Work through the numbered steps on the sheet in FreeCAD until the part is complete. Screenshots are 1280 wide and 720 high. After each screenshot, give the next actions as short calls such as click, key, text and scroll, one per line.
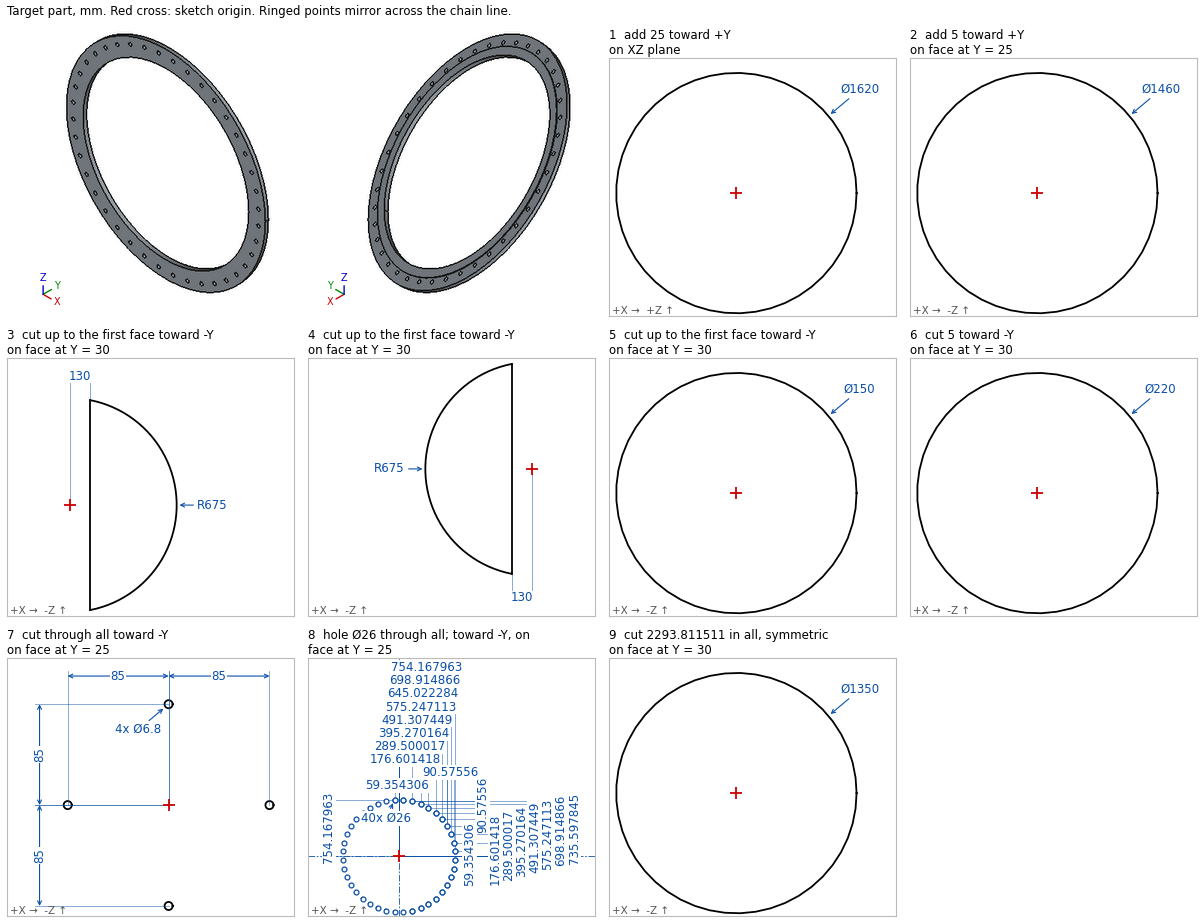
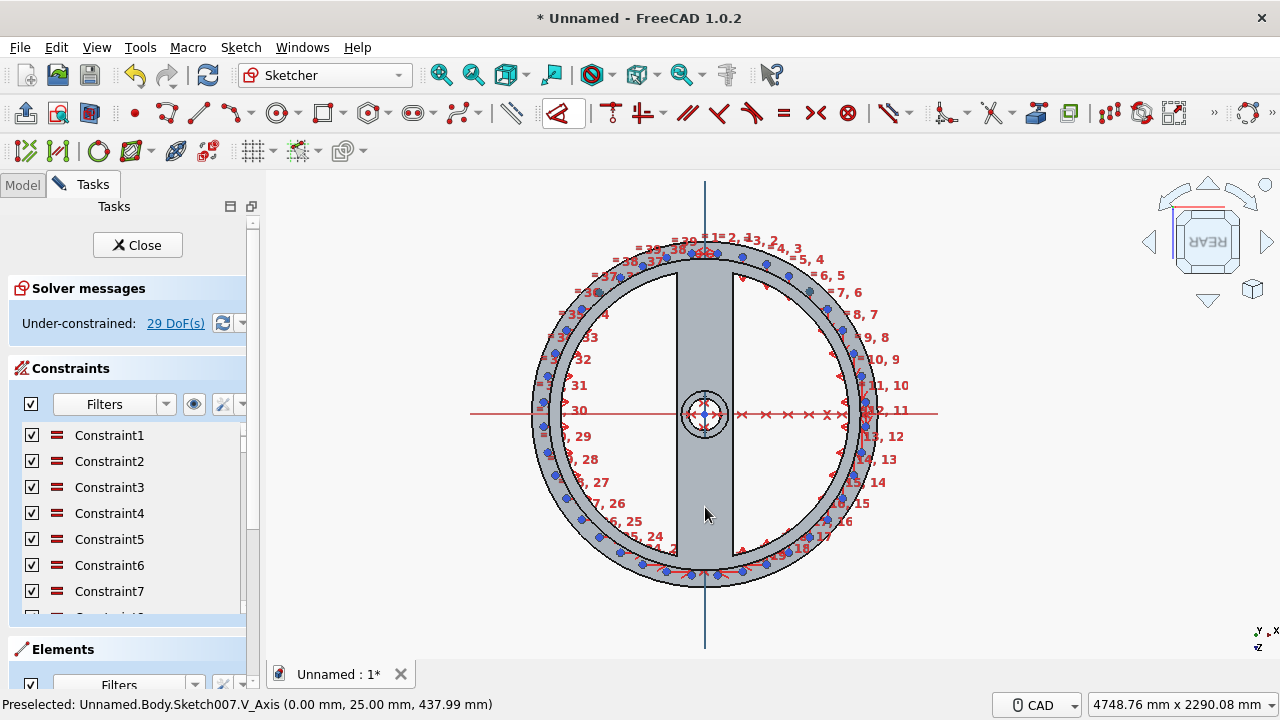
click(816, 114)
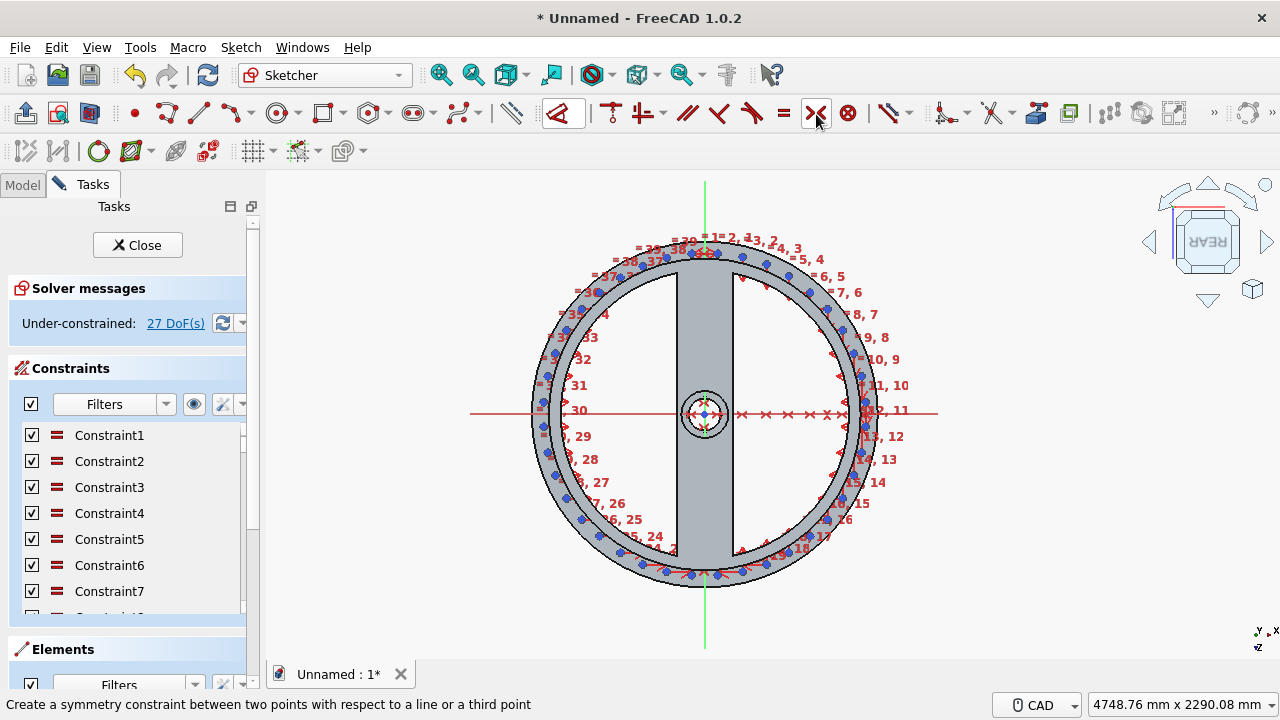
click(789, 276)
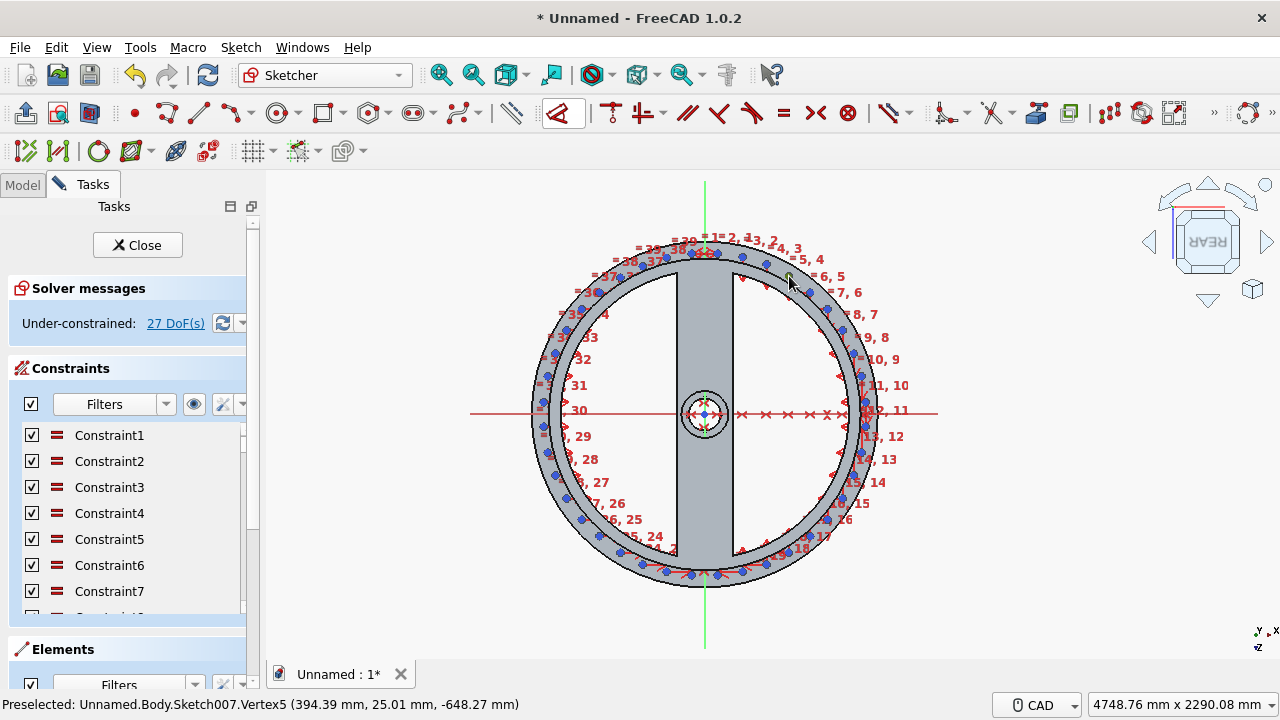
click(620, 278)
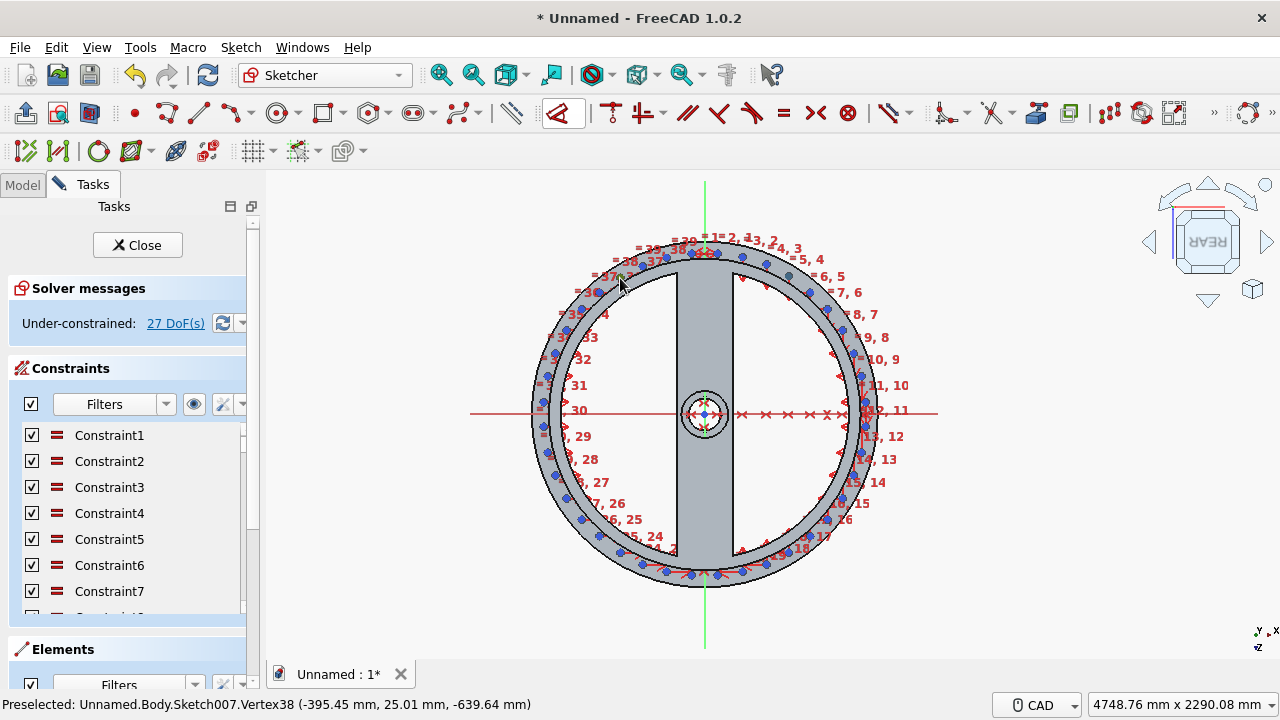
click(705, 507)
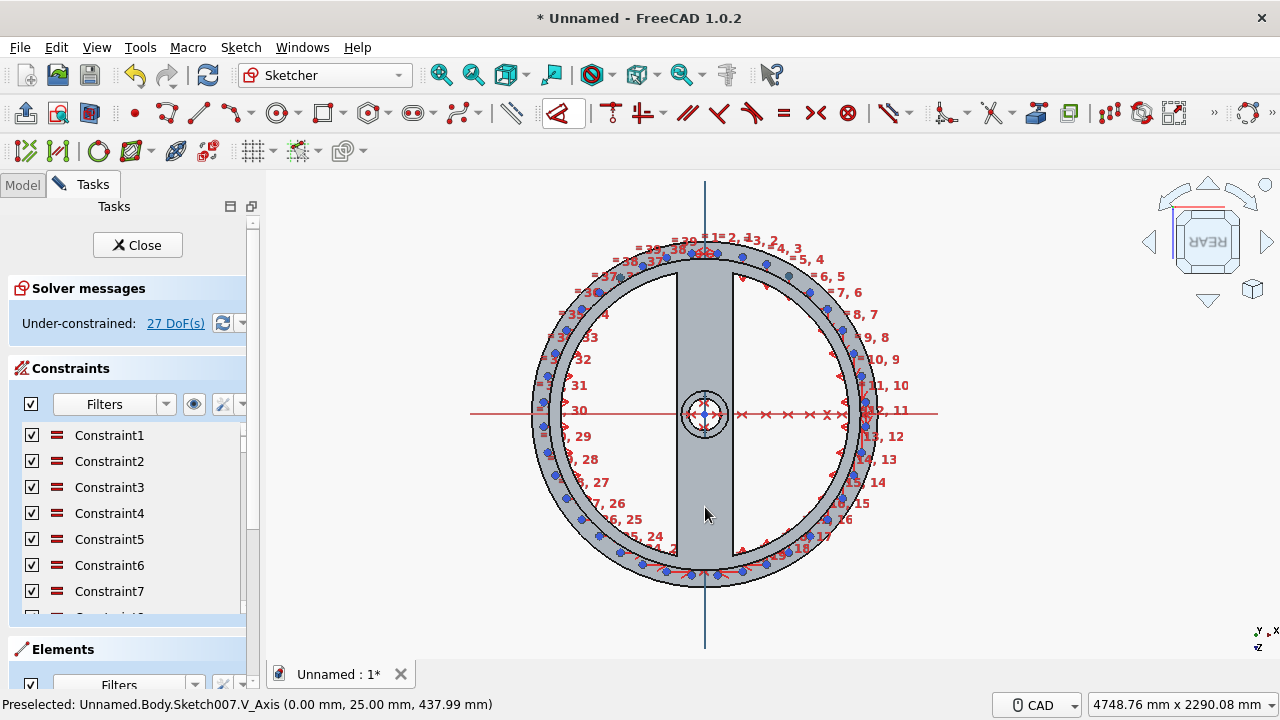
click(816, 114)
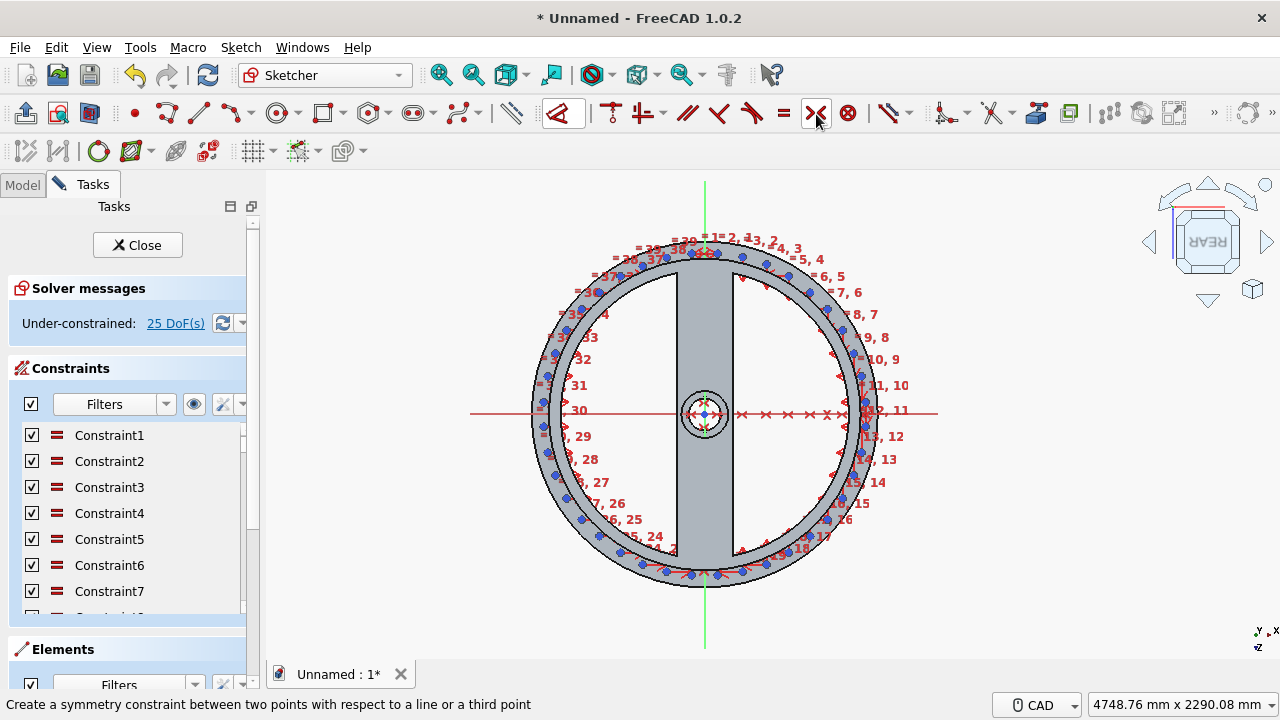
click(767, 264)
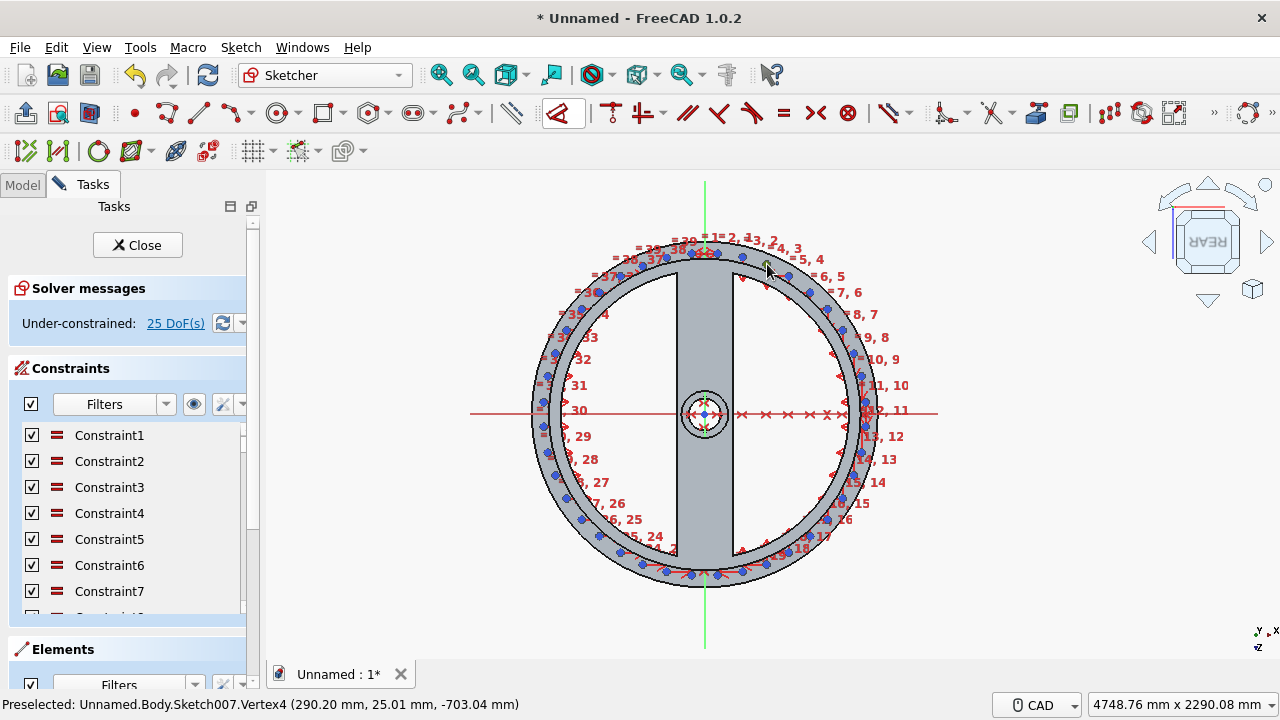
click(643, 266)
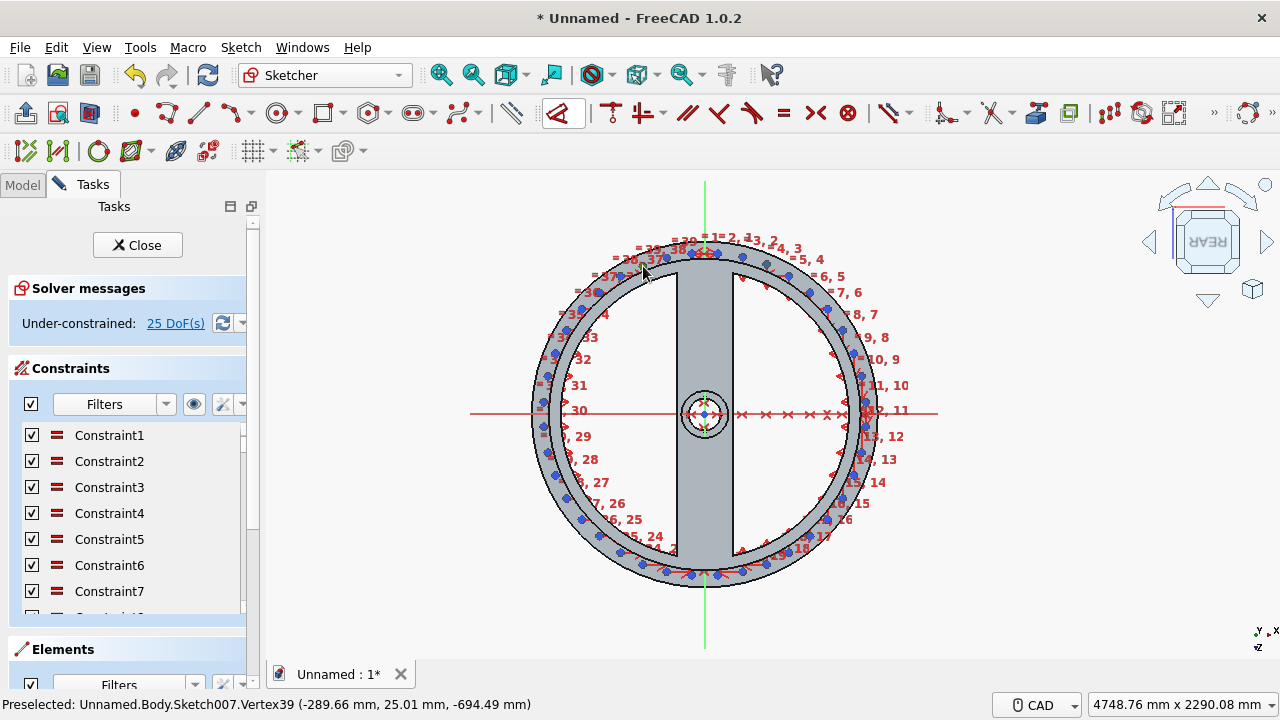
click(705, 507)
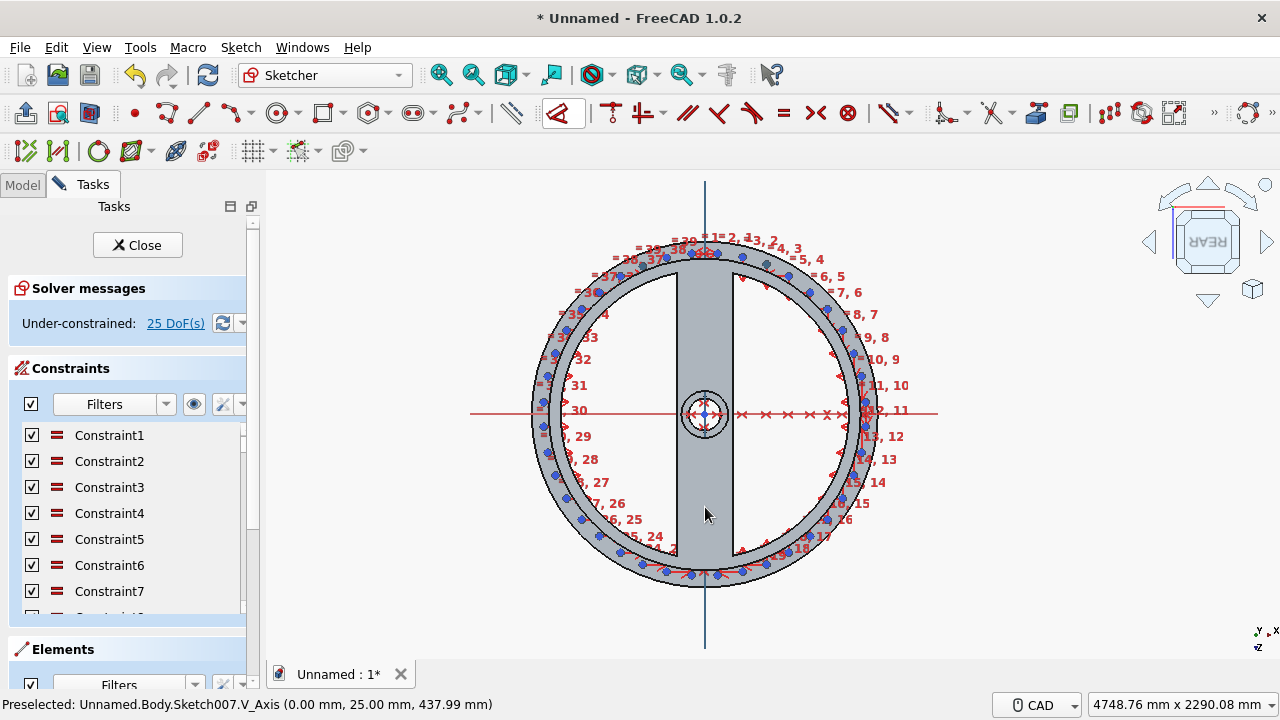
key(s)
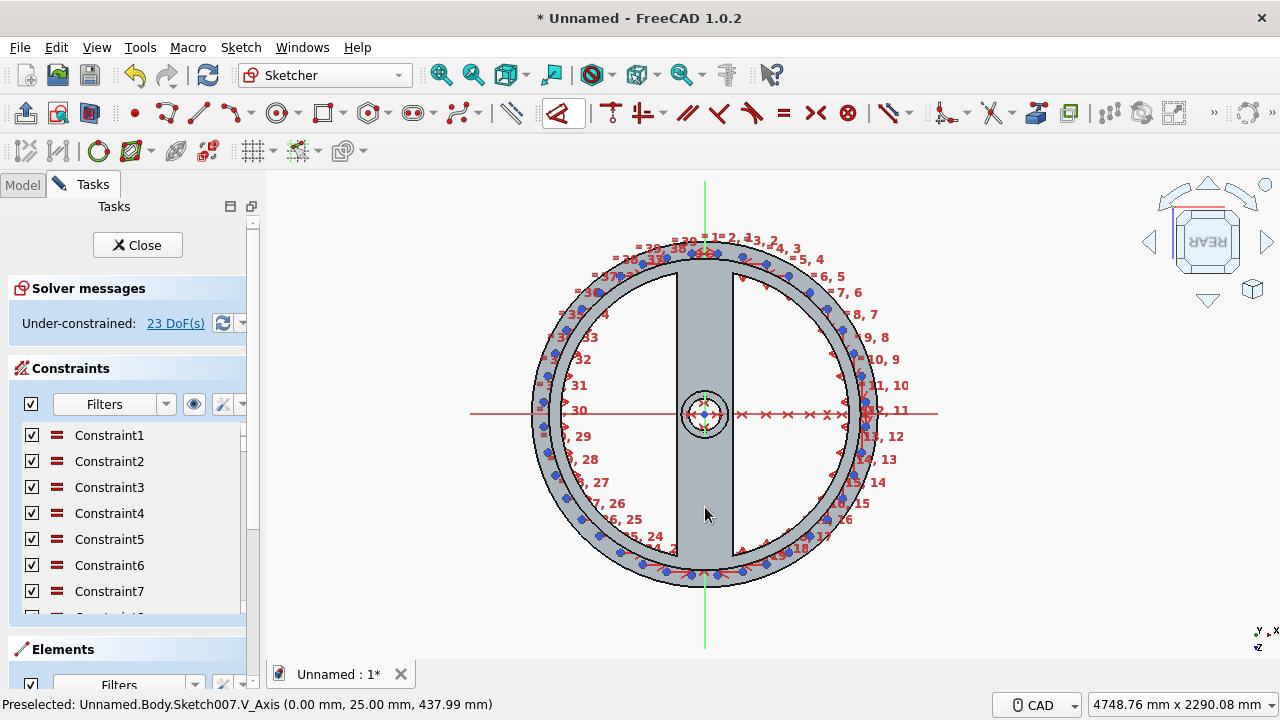
click(743, 257)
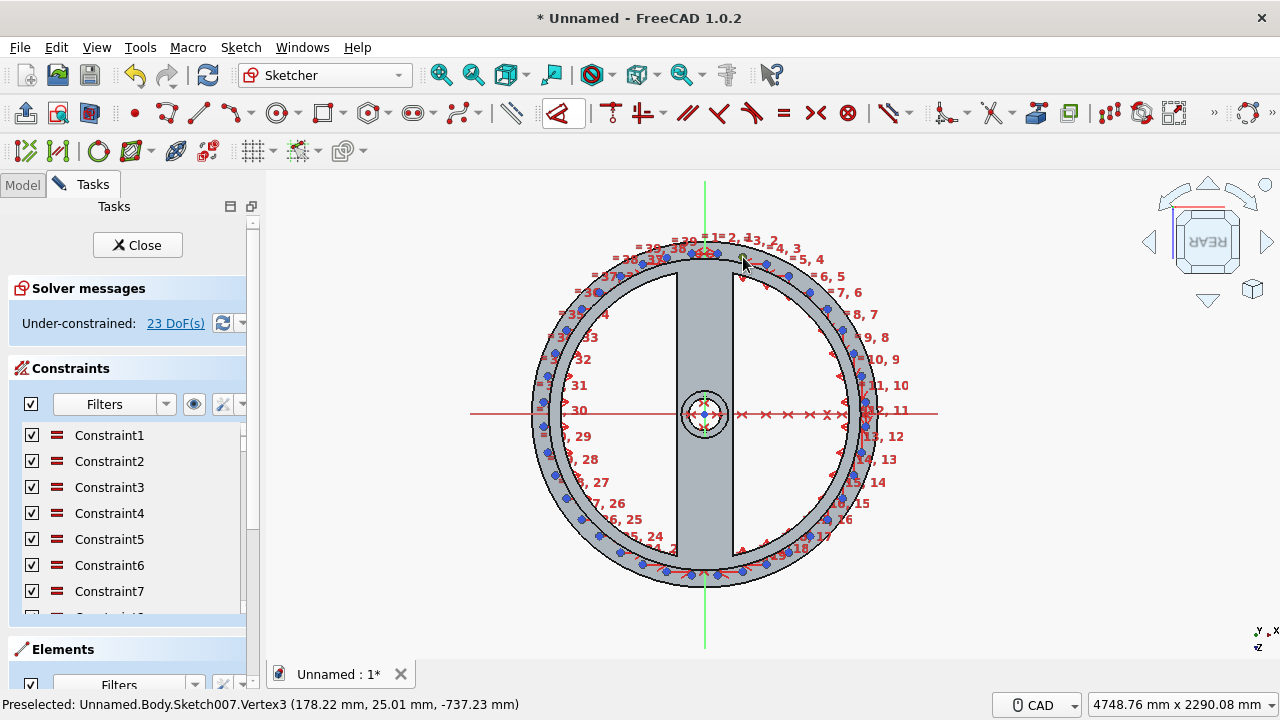
click(667, 258)